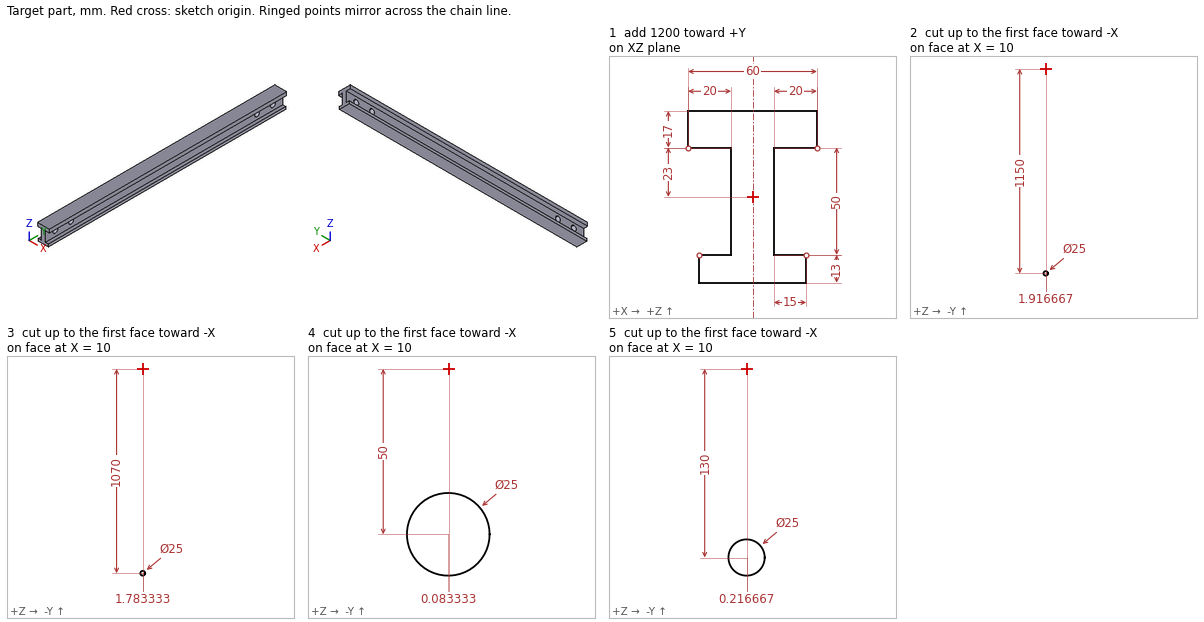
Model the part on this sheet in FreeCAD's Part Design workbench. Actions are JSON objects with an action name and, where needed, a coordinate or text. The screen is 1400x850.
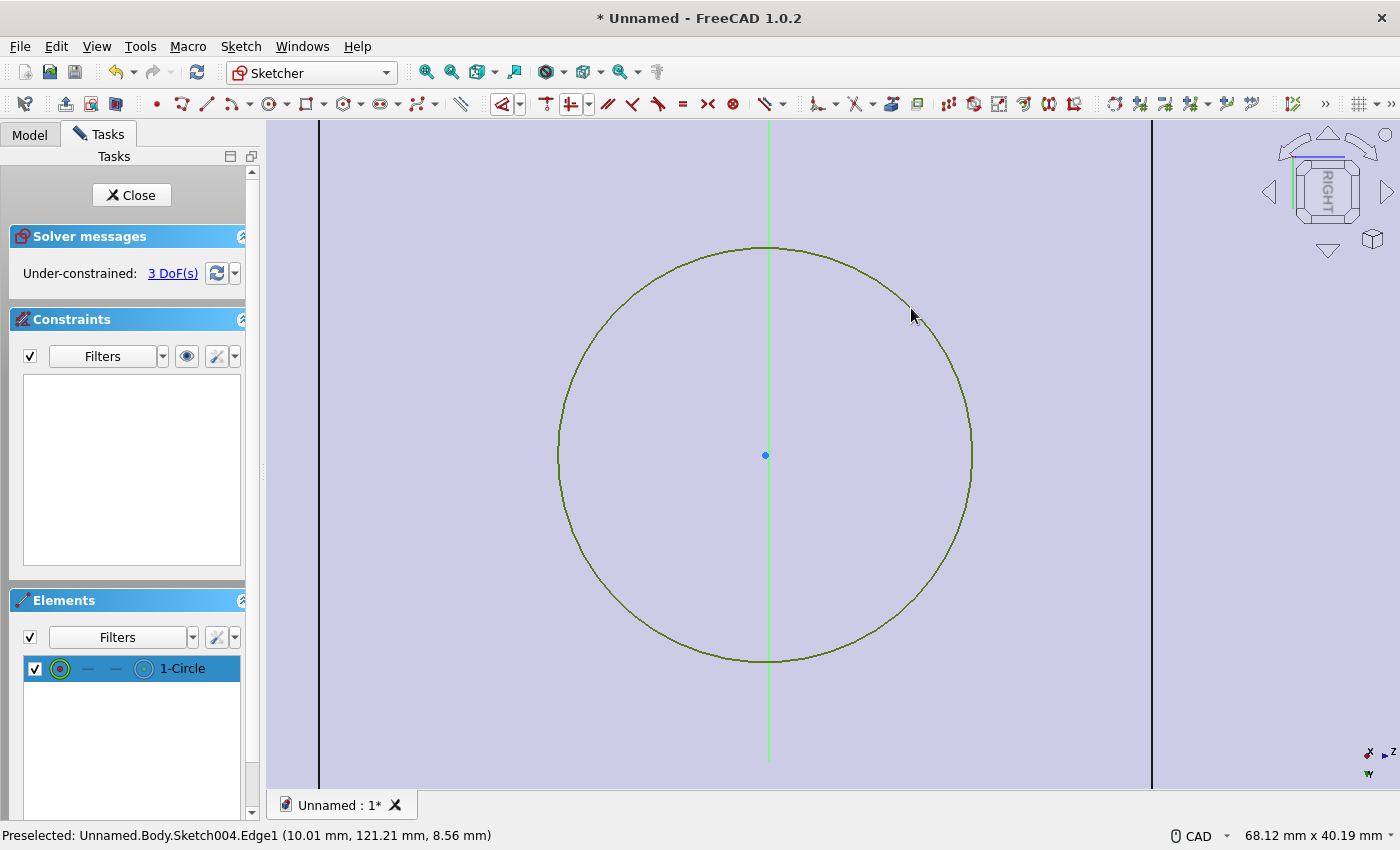
{"action": "key", "text": "k o"}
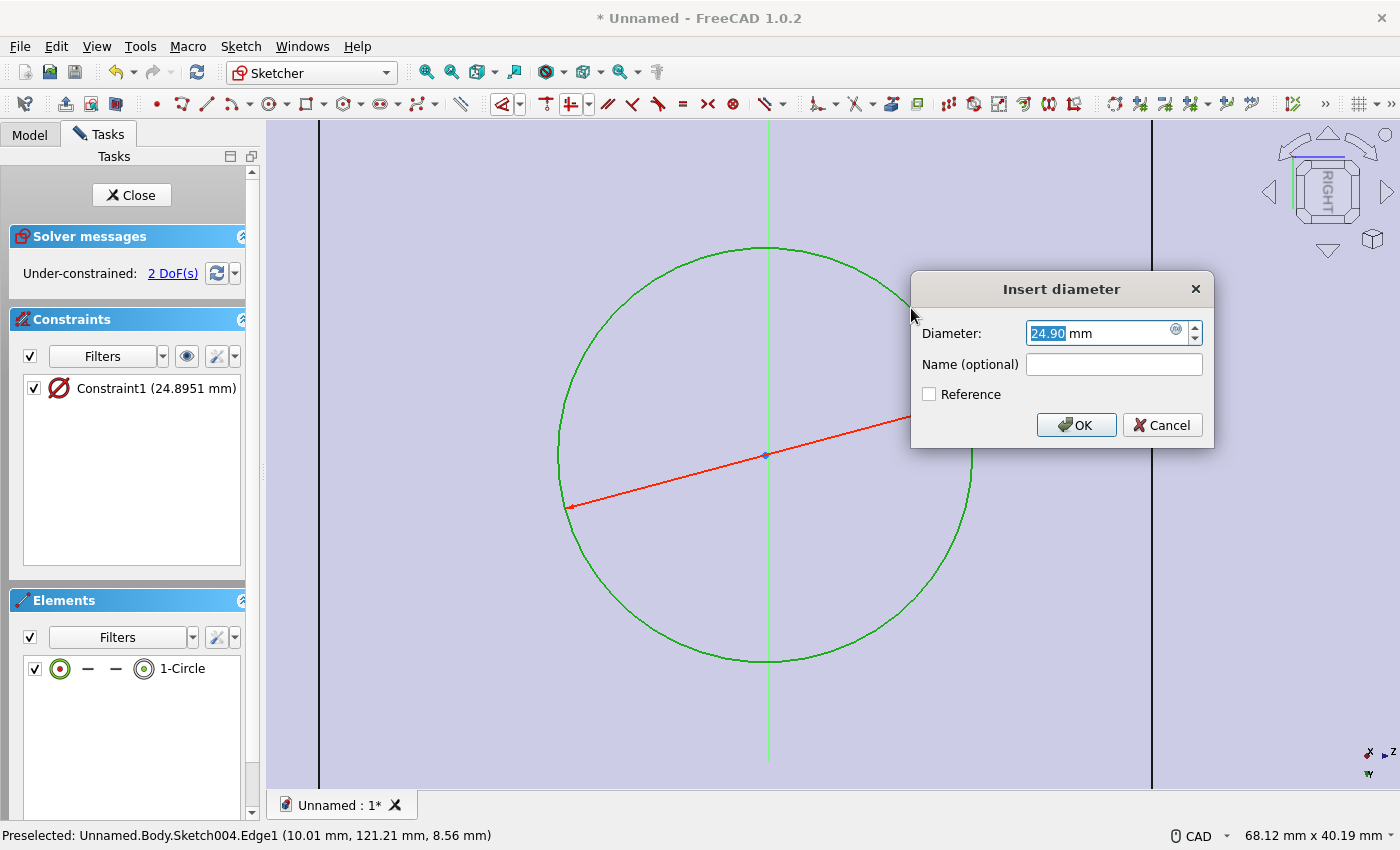
{"action": "type", "text": "25"}
{"action": "key", "text": "Return"}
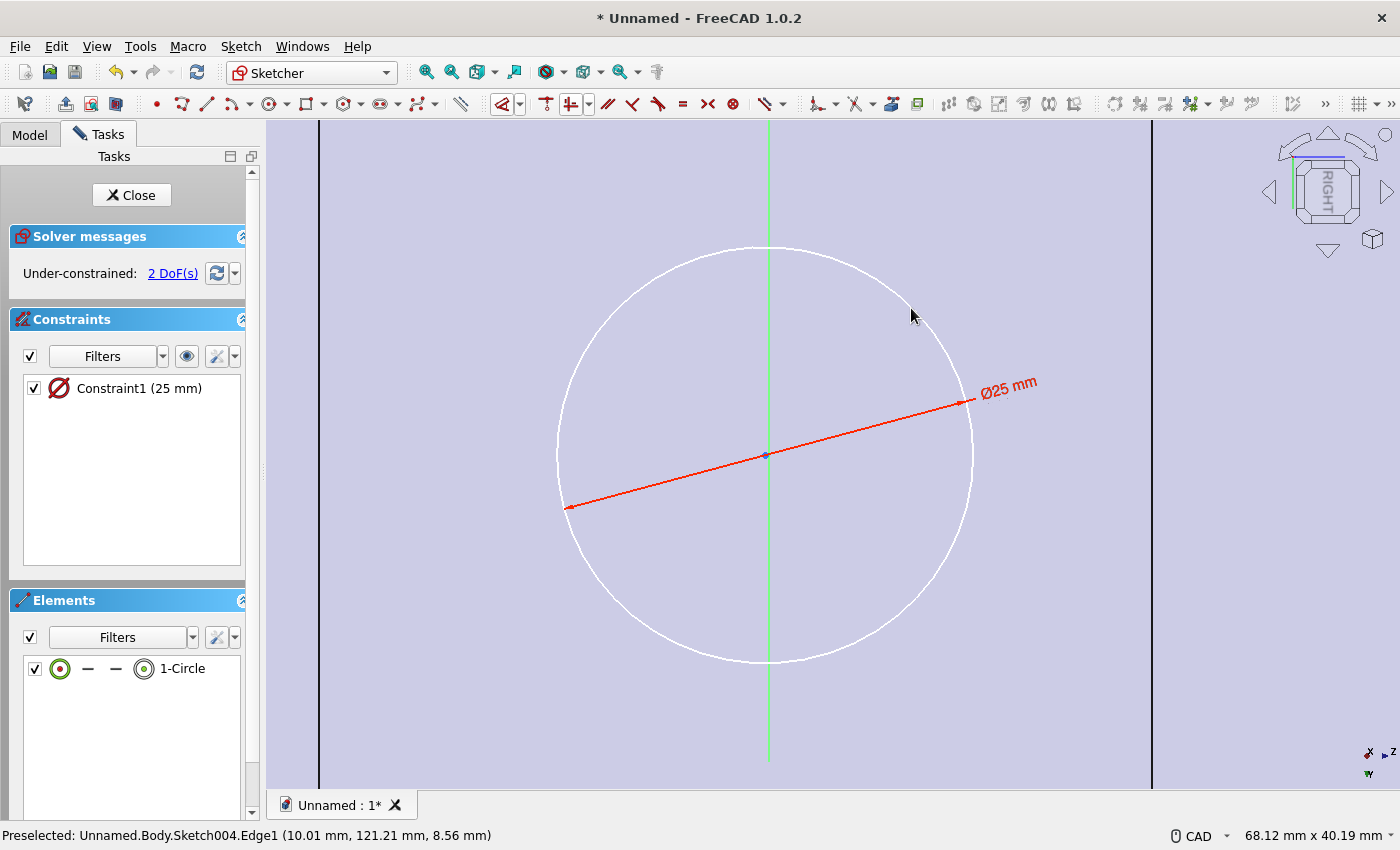
{"action": "left_click", "coordinate": [765, 455]}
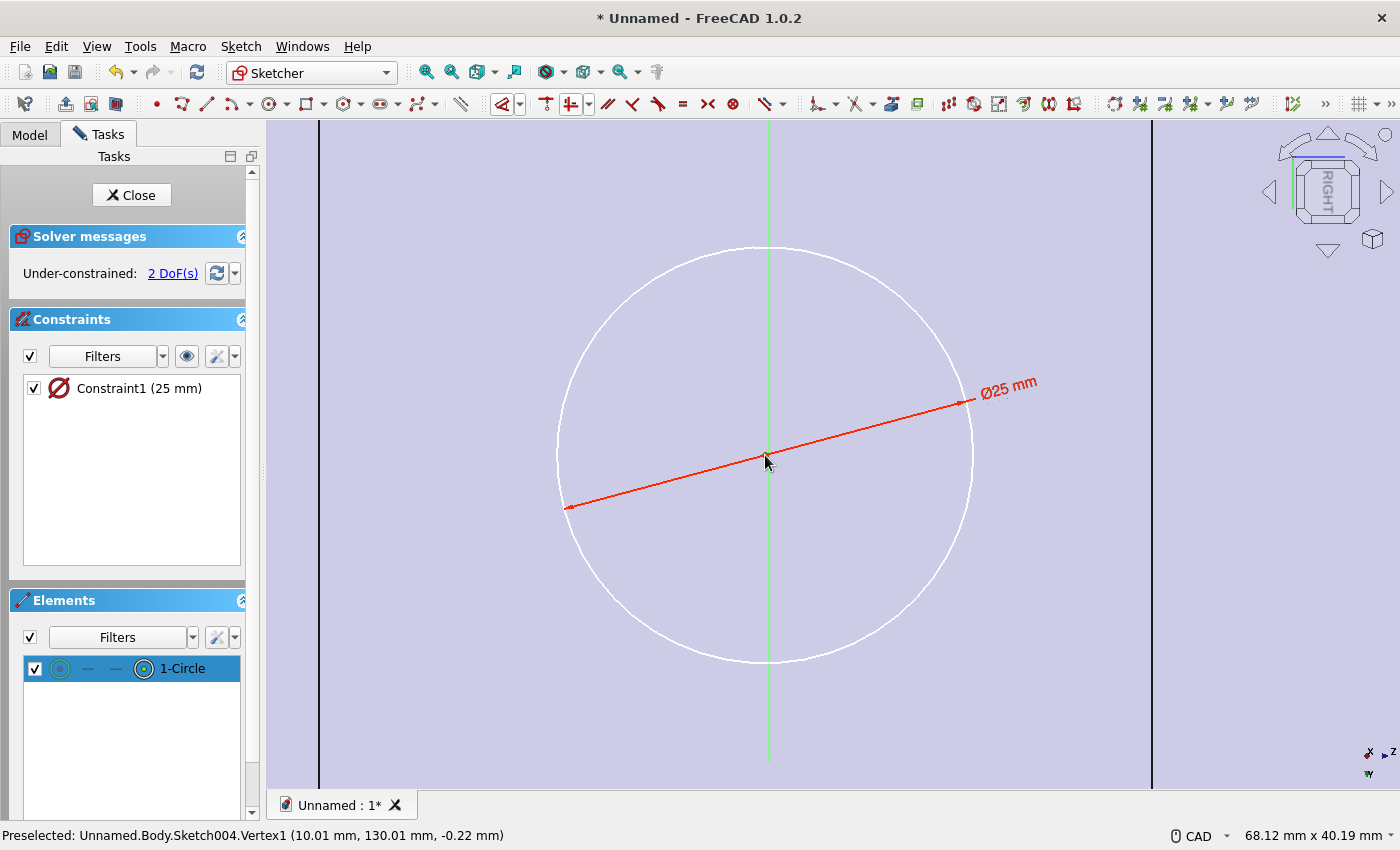
{"action": "left_click", "coordinate": [520, 104]}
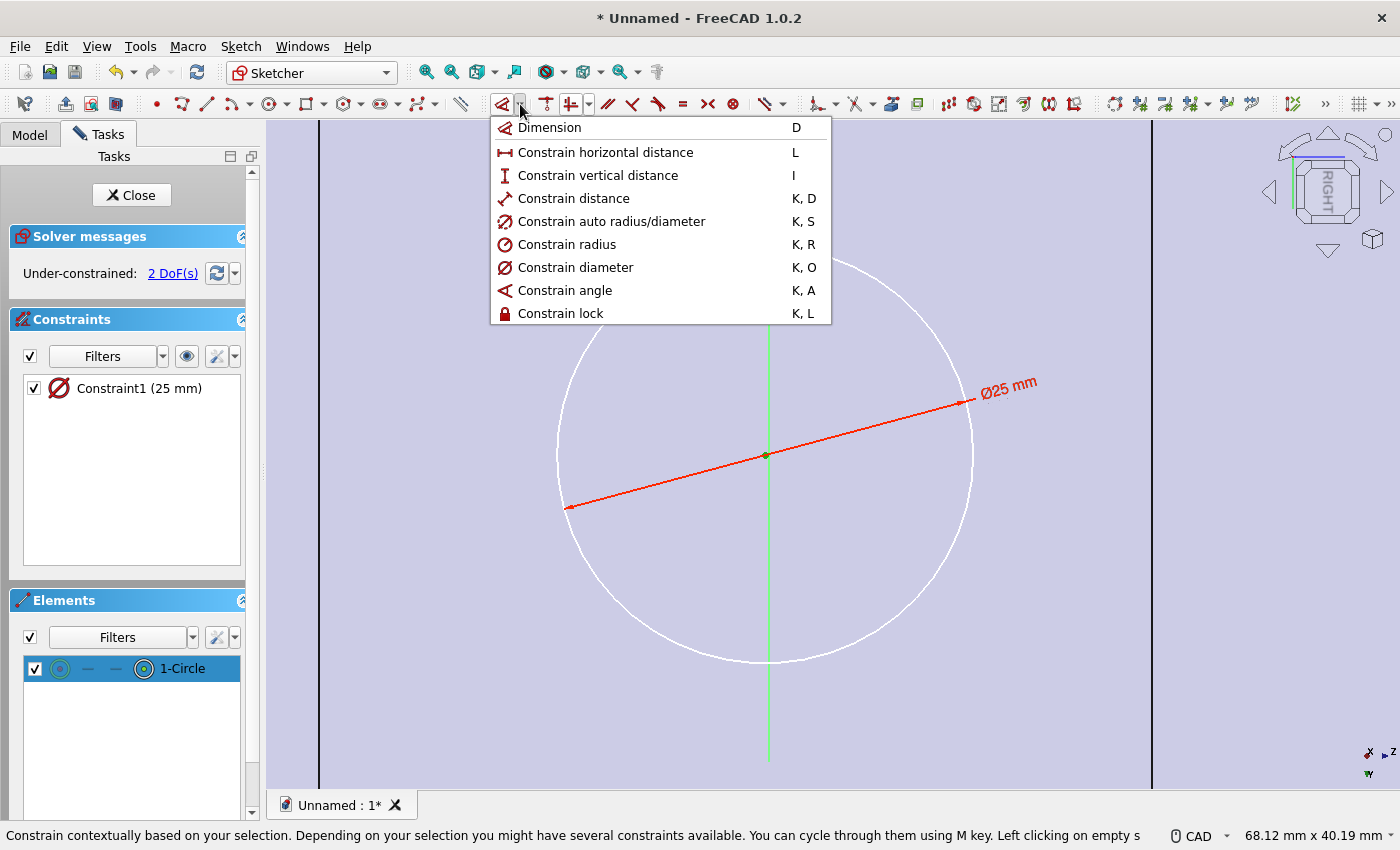
{"action": "left_click", "coordinate": [661, 176]}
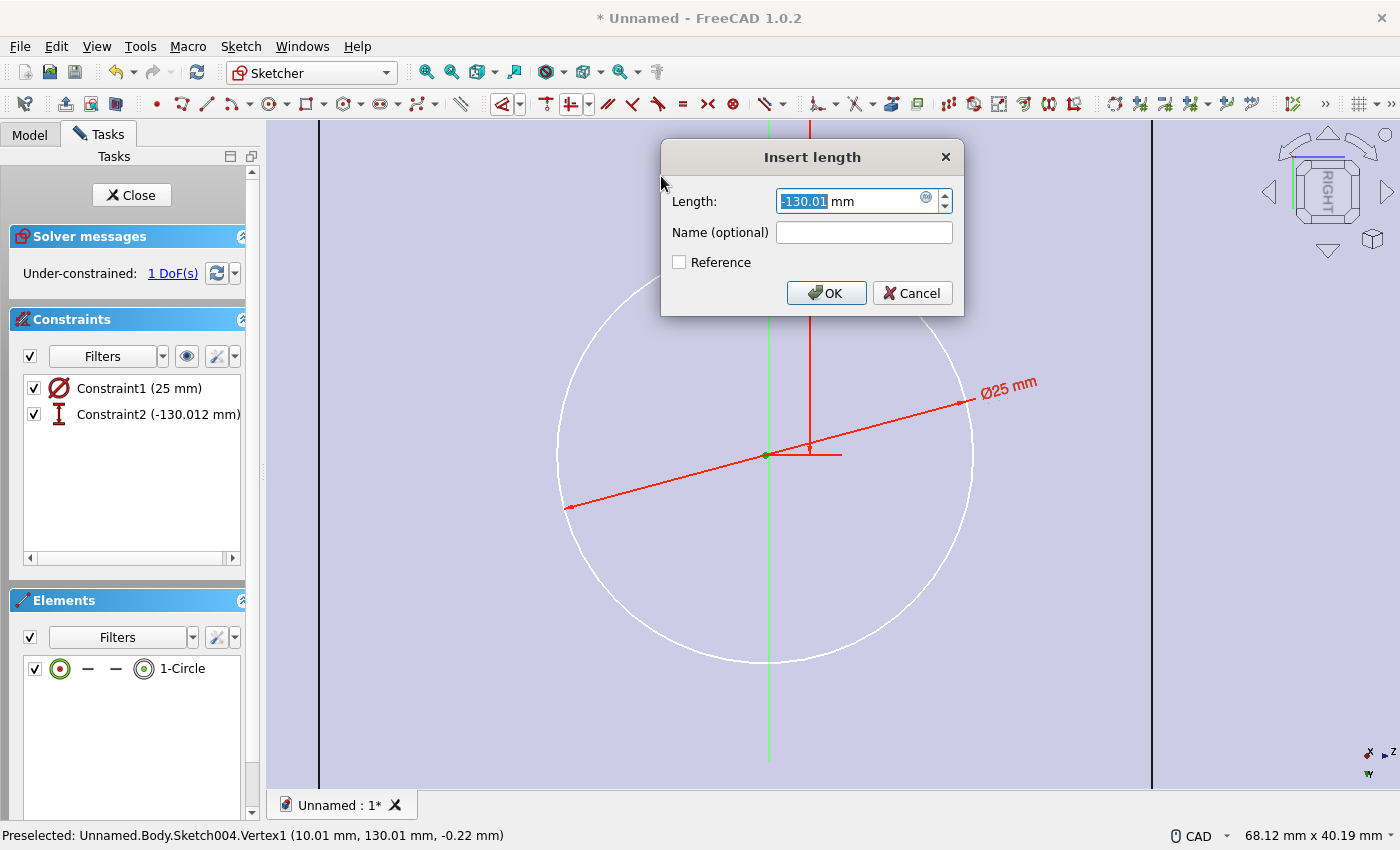
{"action": "type", "text": "-130"}
{"action": "key", "text": "Return"}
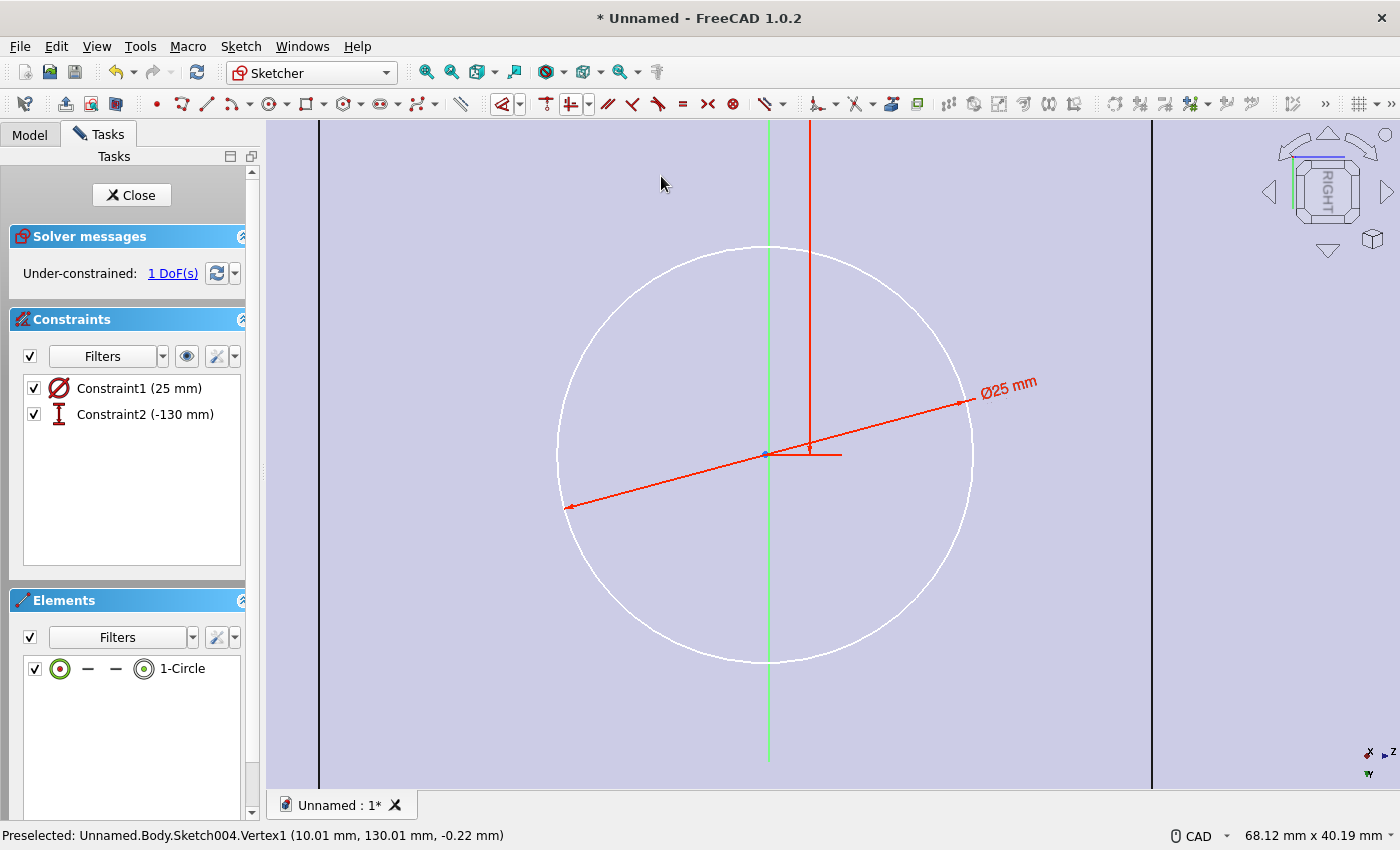
{"action": "scroll", "coordinate": [765, 455], "scroll_direction": "up", "scroll_amount": 12}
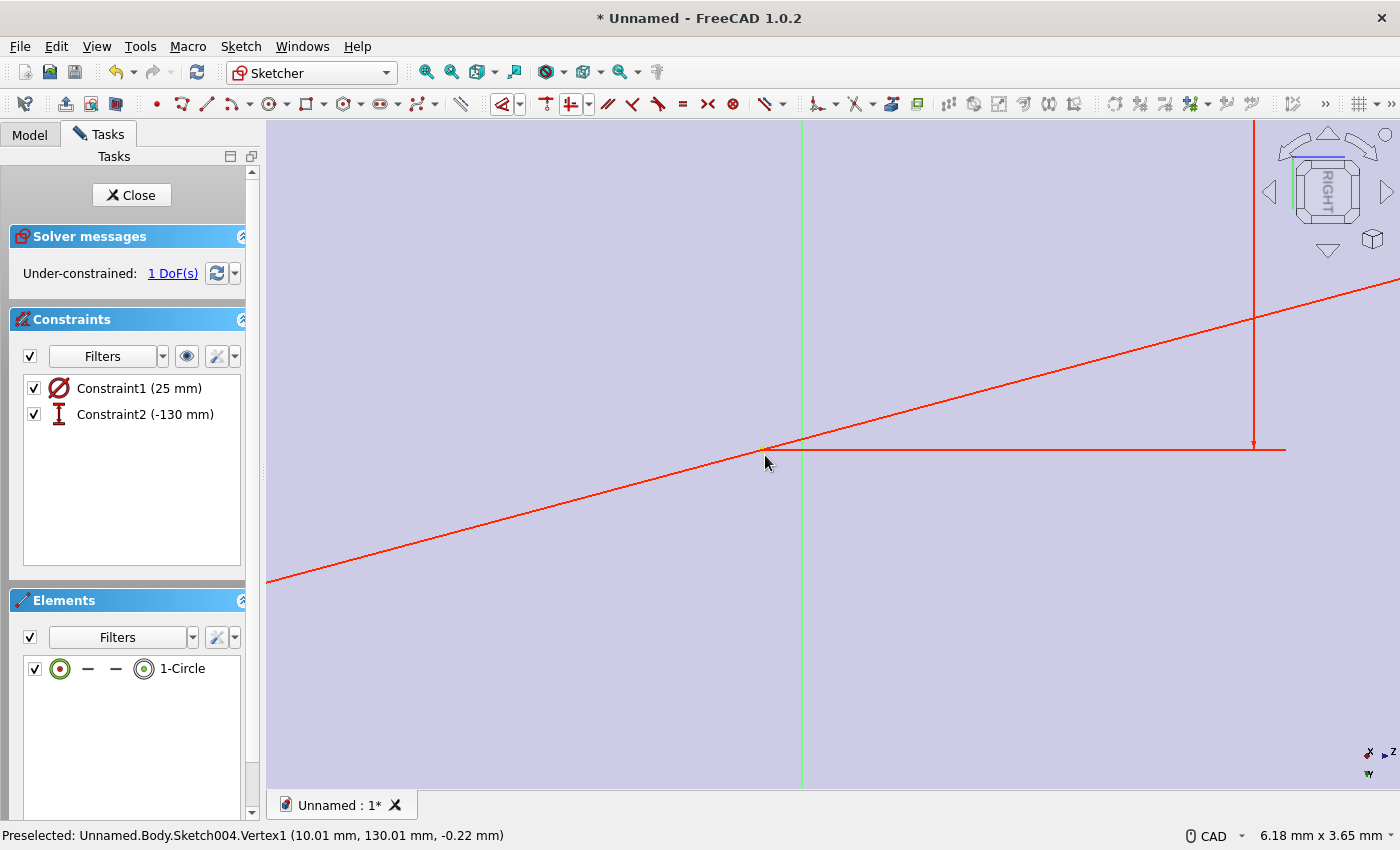
{"action": "left_click", "coordinate": [762, 450]}